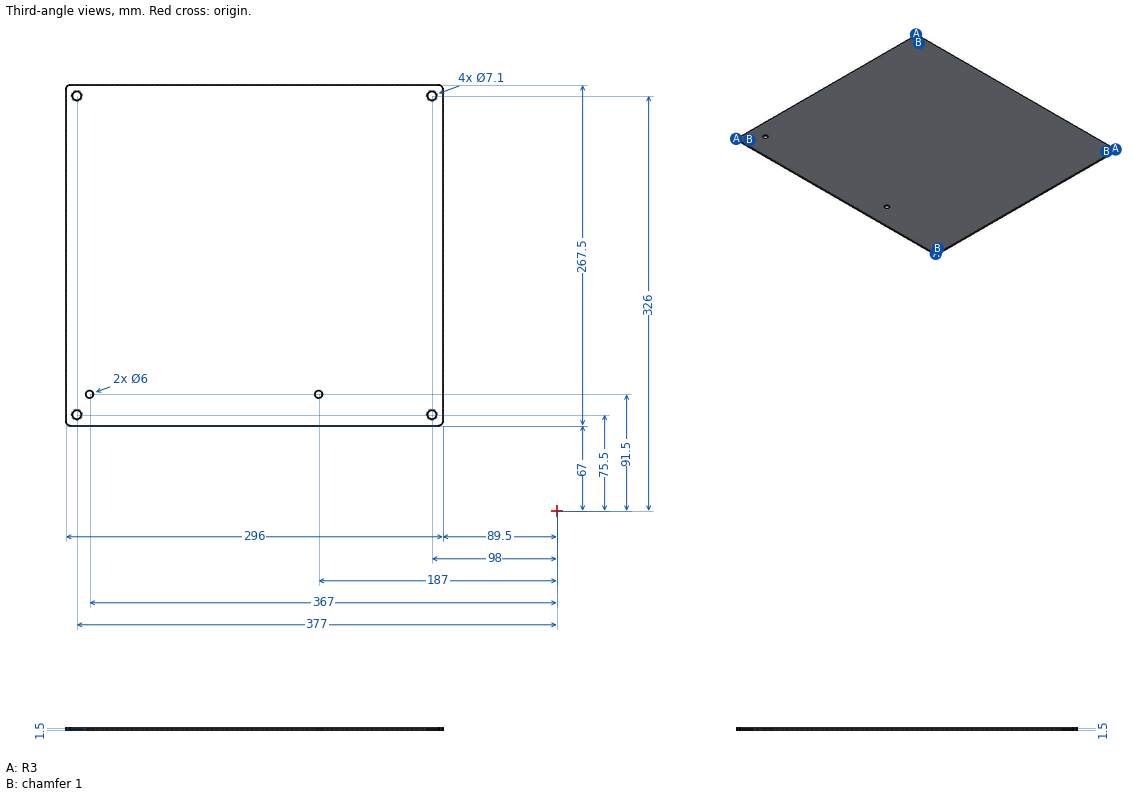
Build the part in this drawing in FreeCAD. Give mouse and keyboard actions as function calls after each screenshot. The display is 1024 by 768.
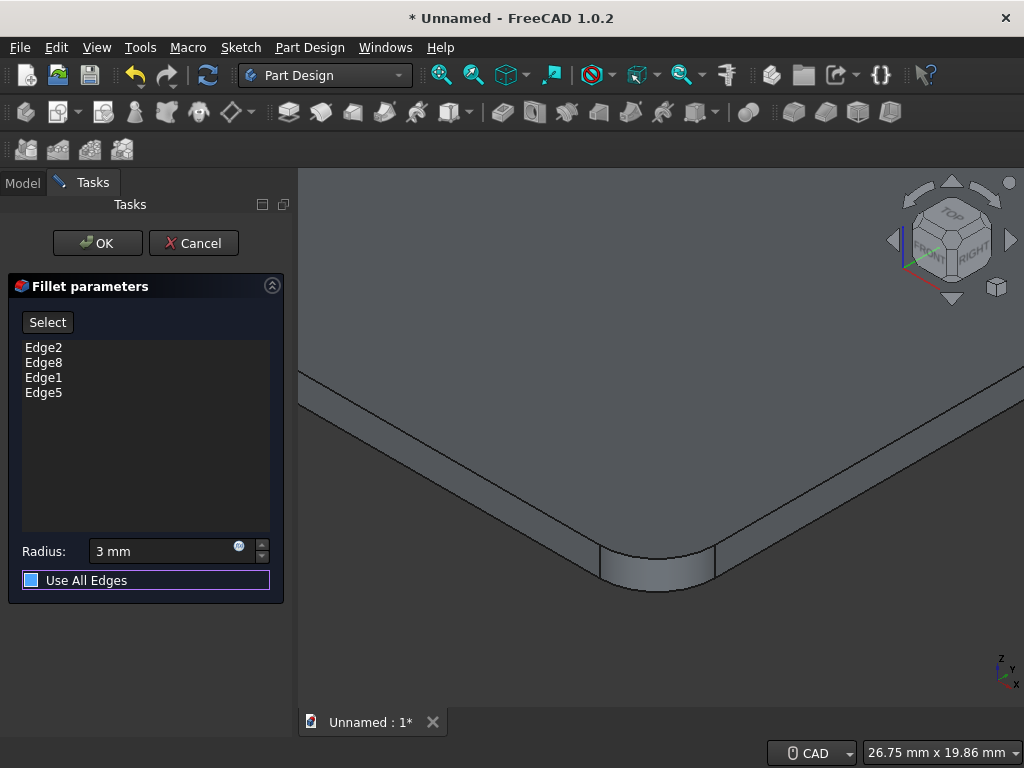
click(98, 243)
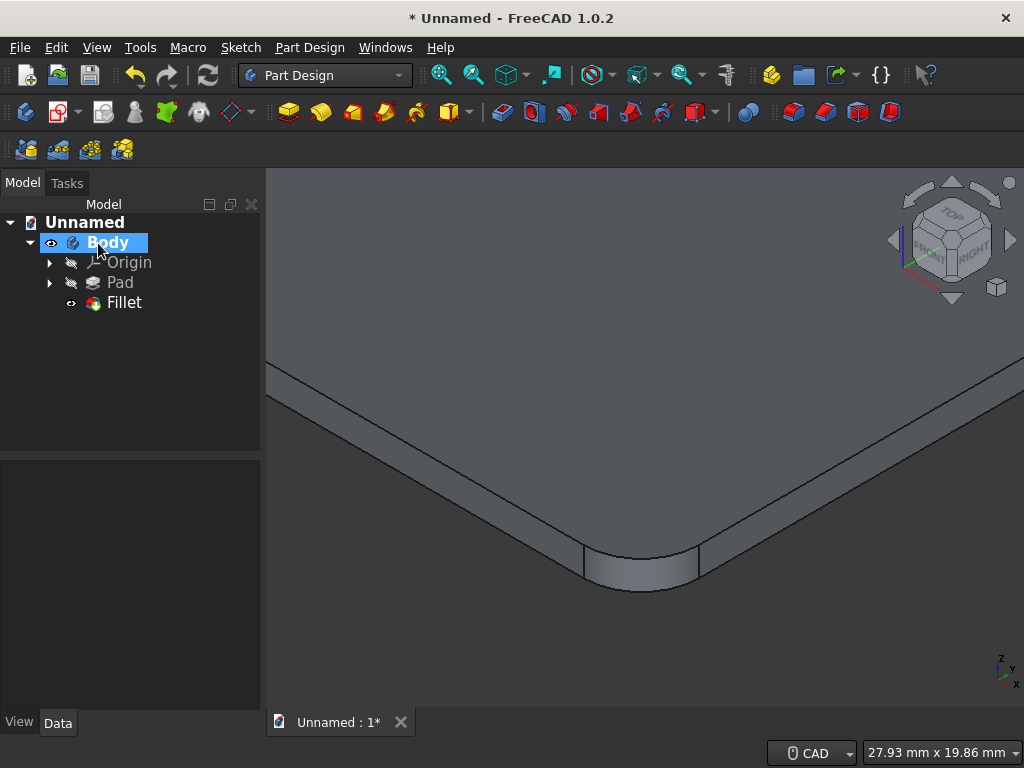
click(442, 76)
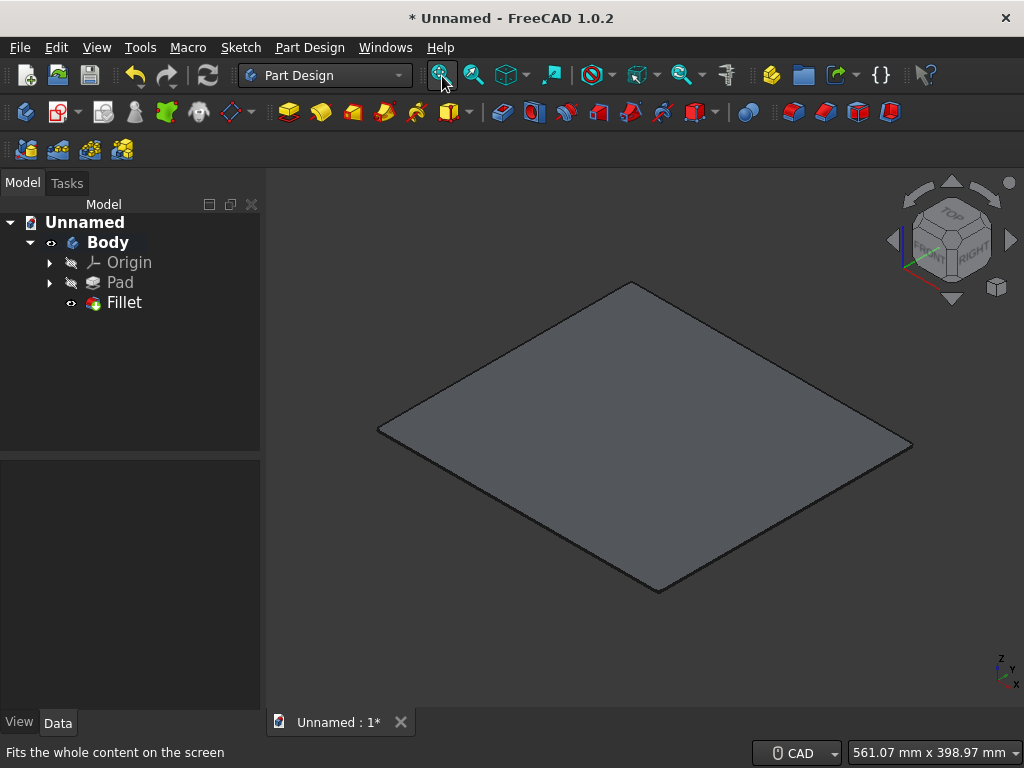
click(58, 112)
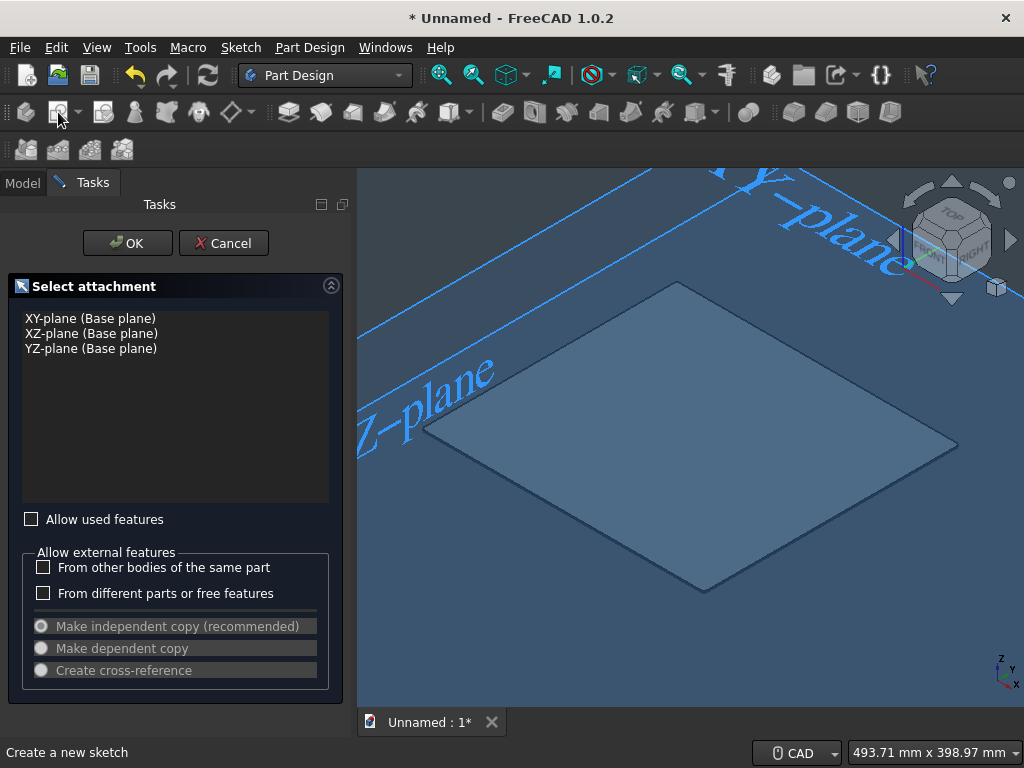
click(82, 318)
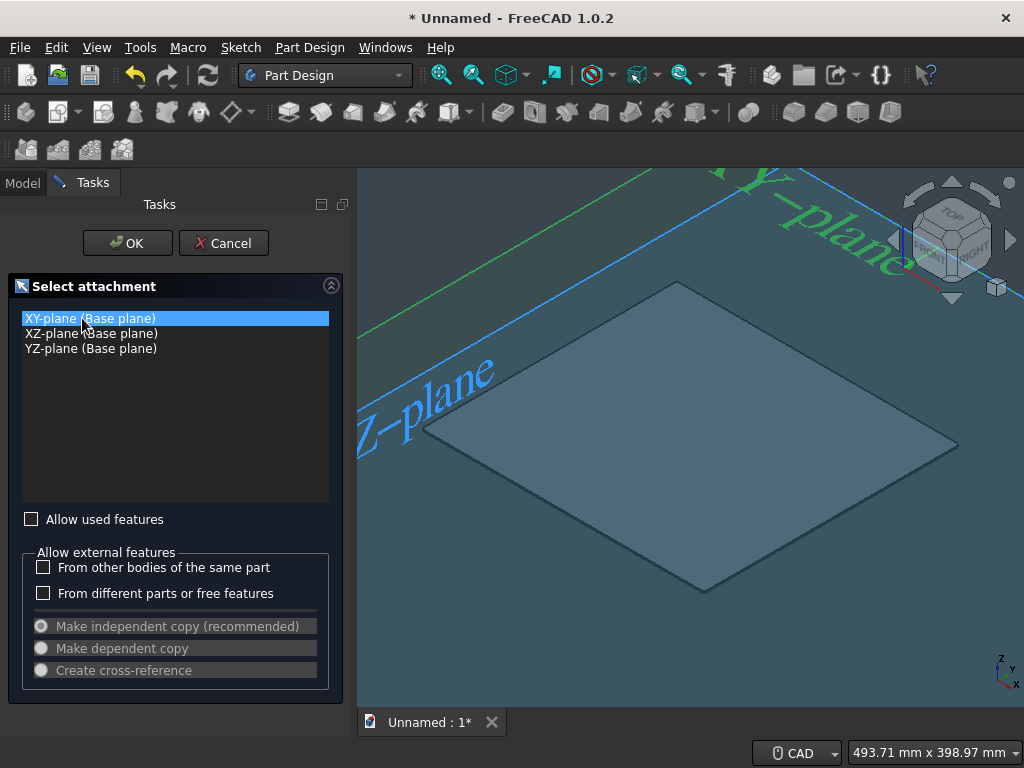
click(128, 243)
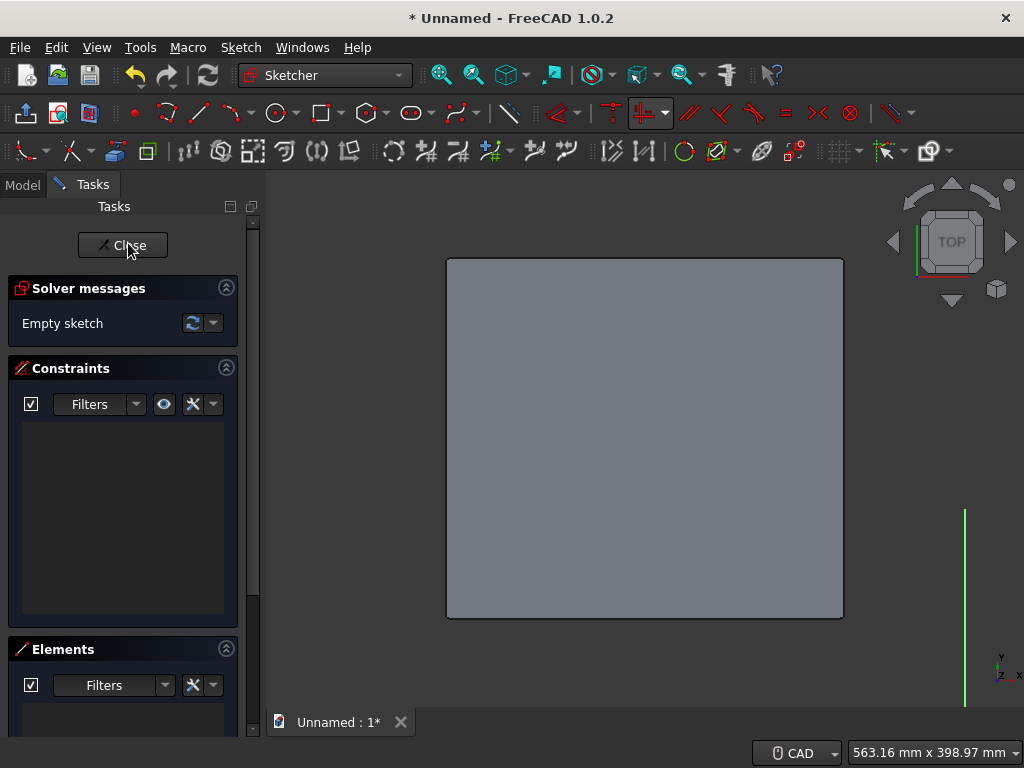
scroll(294, 198, down, 2)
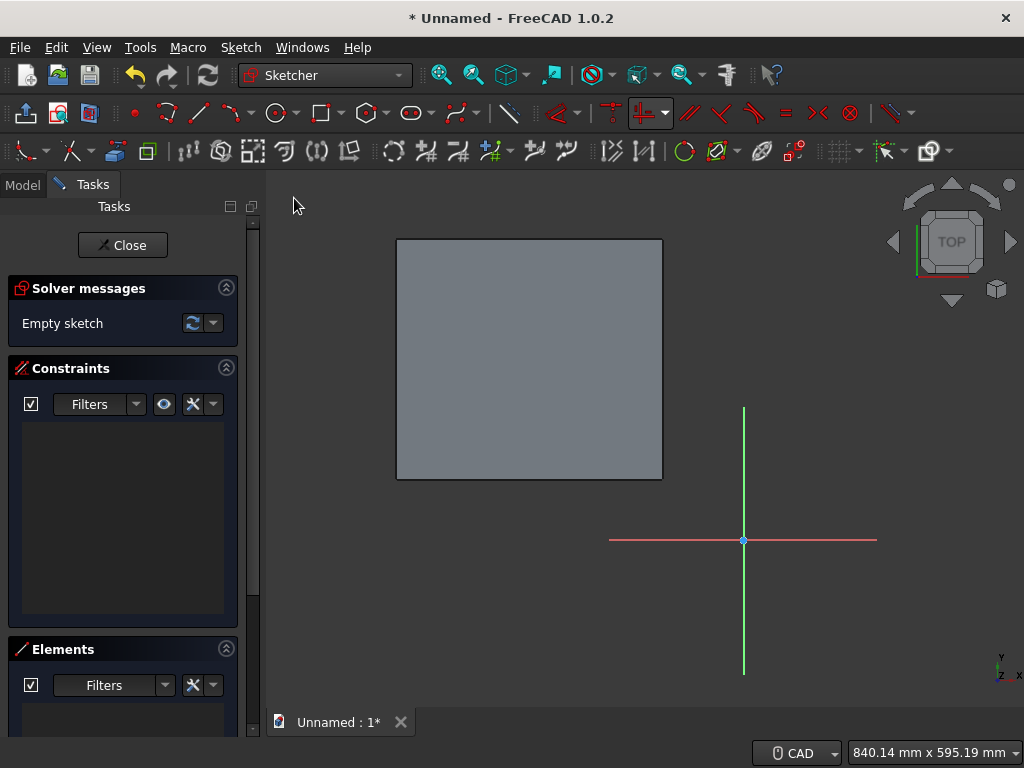
click(276, 114)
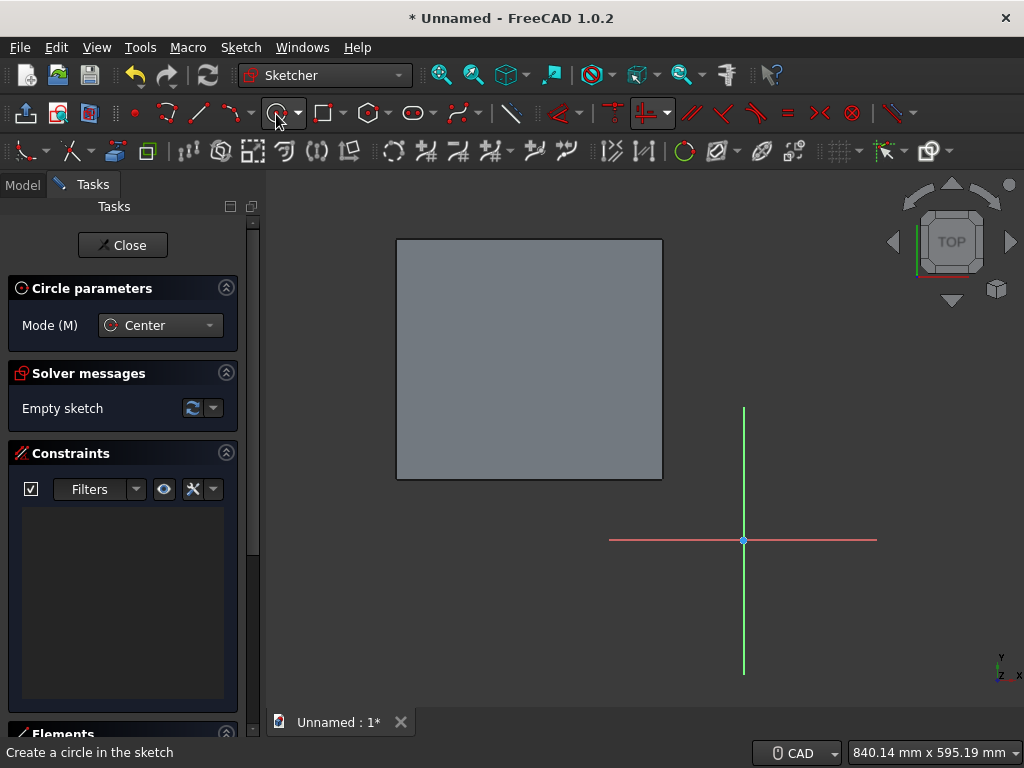
scroll(412, 458, up, 11)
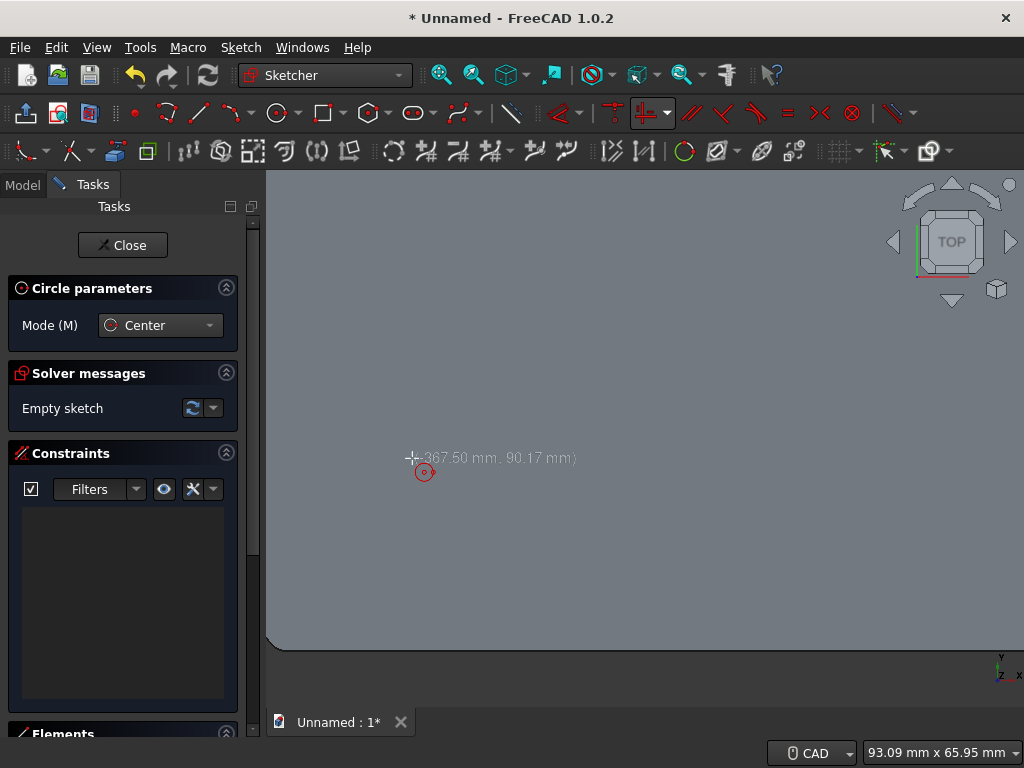
scroll(370, 380, down, 10)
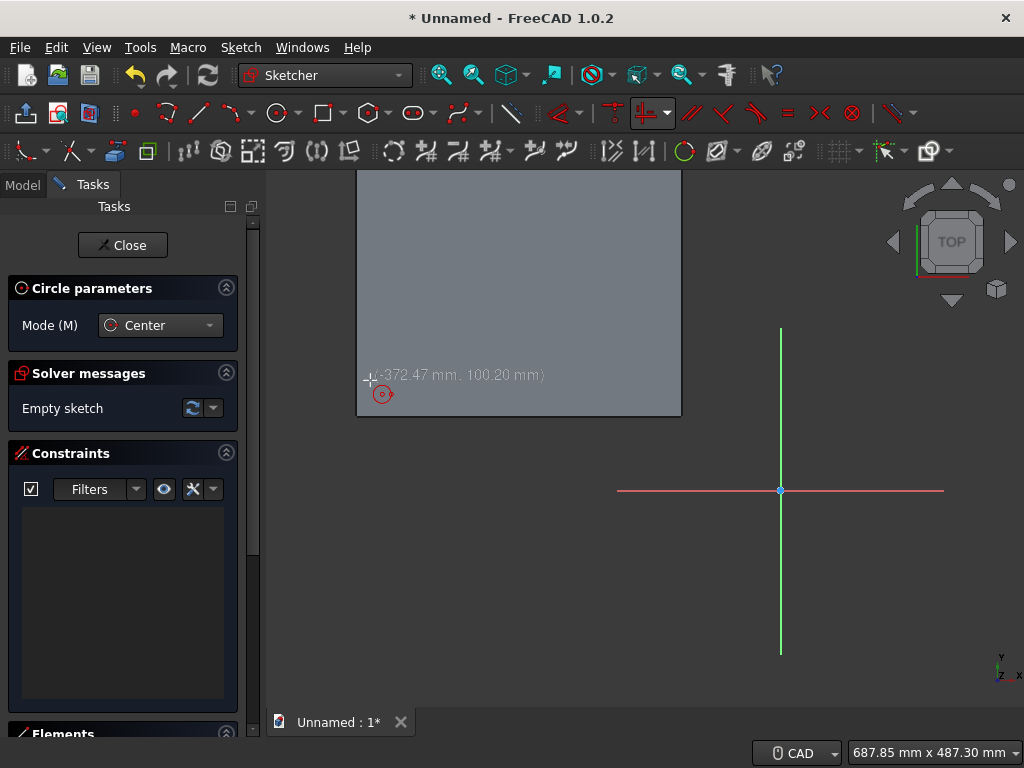
click(376, 390)
move(378, 388)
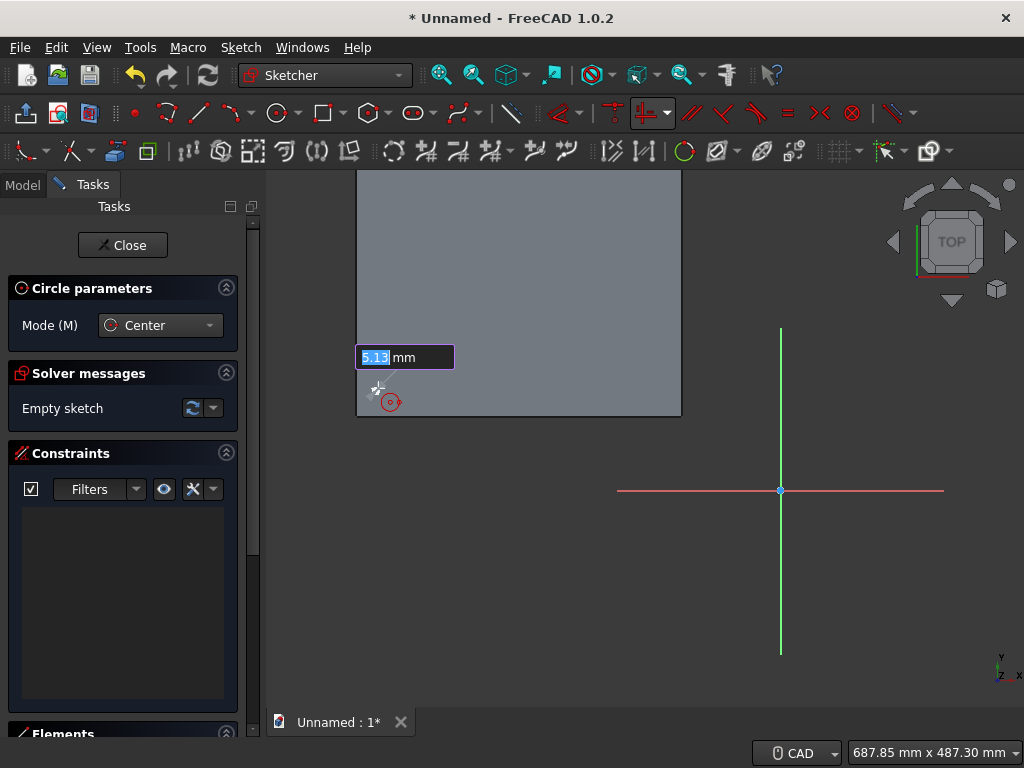
text(6)
key(Return)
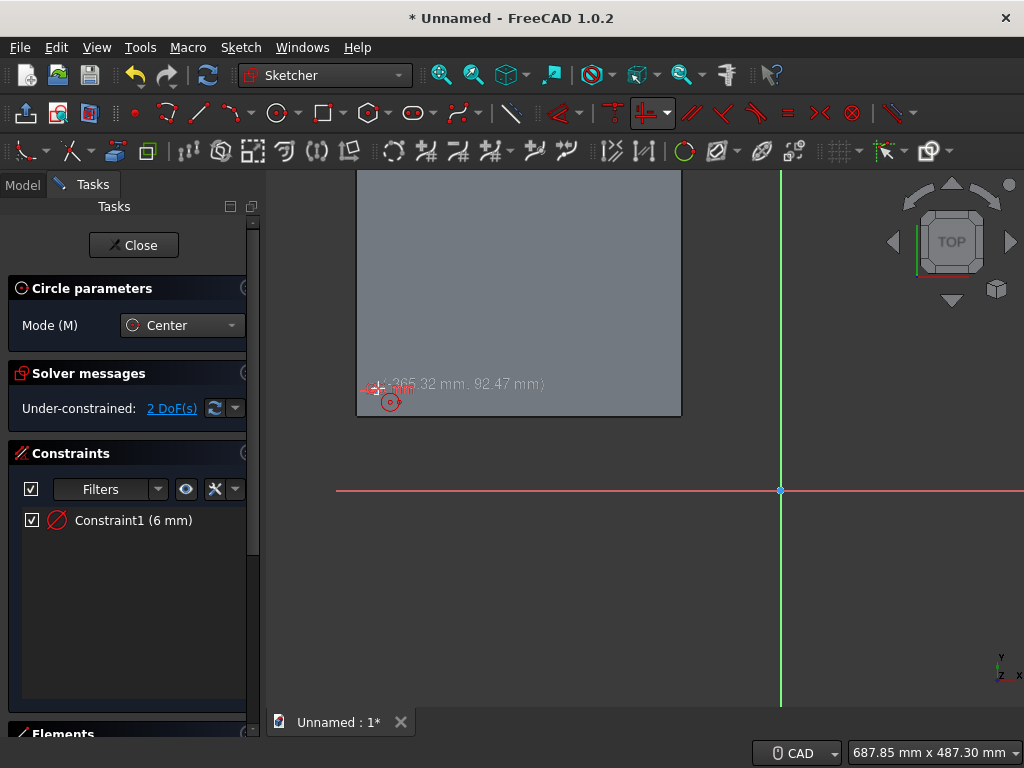
scroll(575, 390, up, 10)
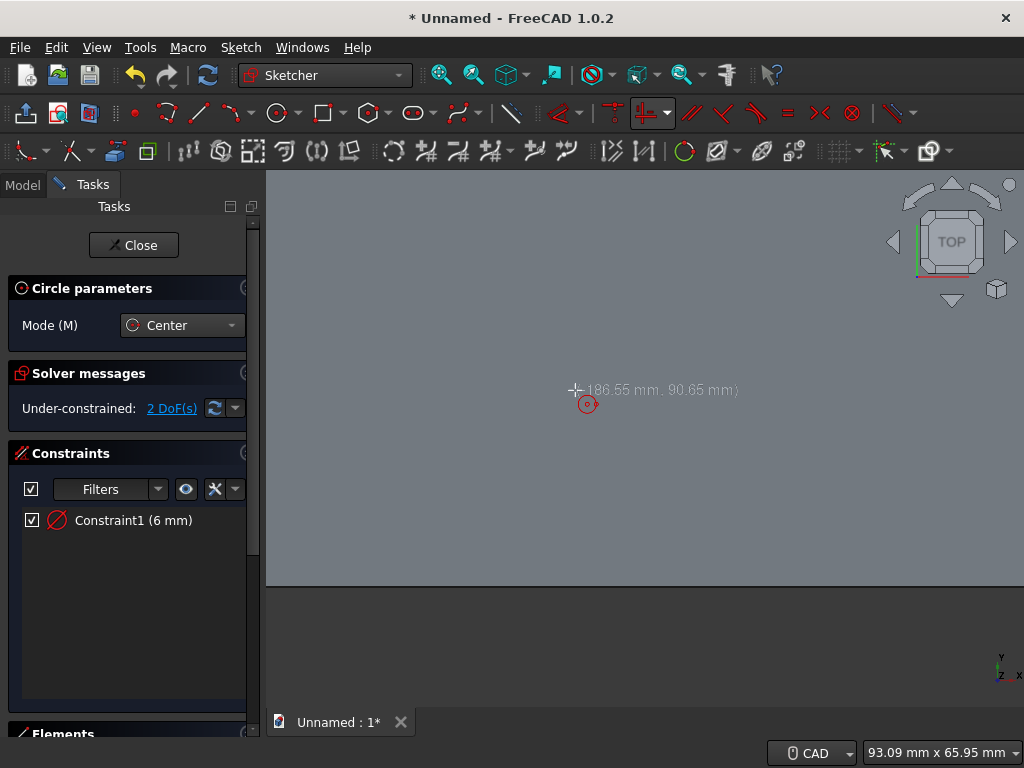
scroll(575, 390, down, 10)